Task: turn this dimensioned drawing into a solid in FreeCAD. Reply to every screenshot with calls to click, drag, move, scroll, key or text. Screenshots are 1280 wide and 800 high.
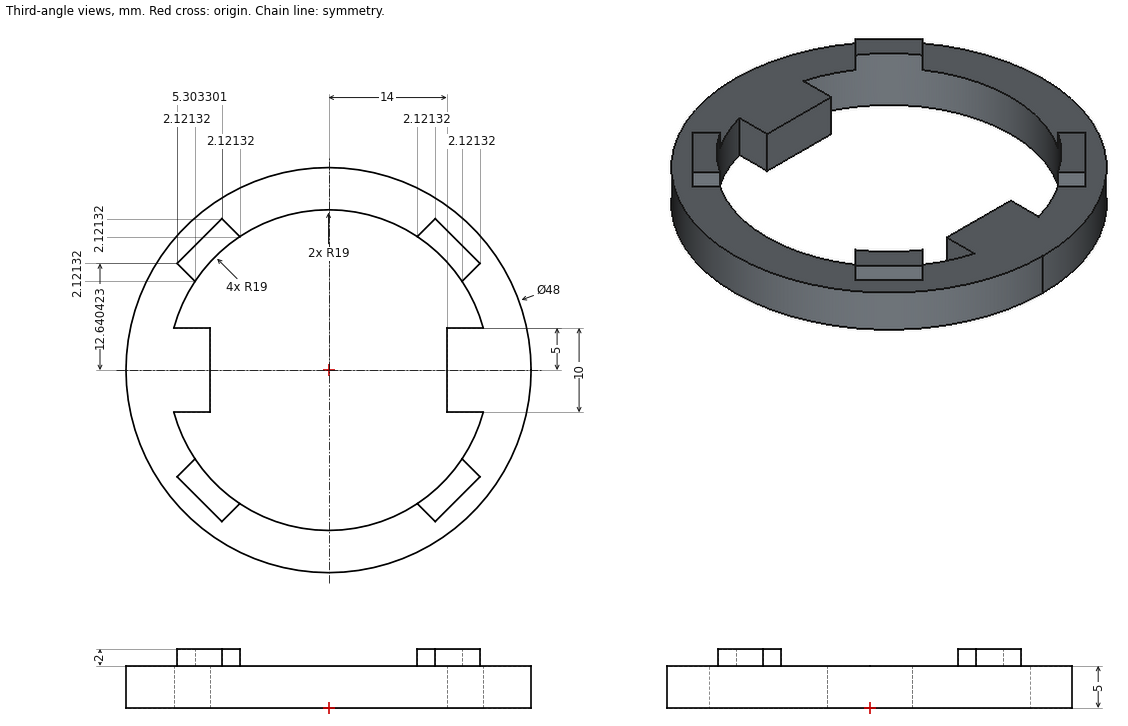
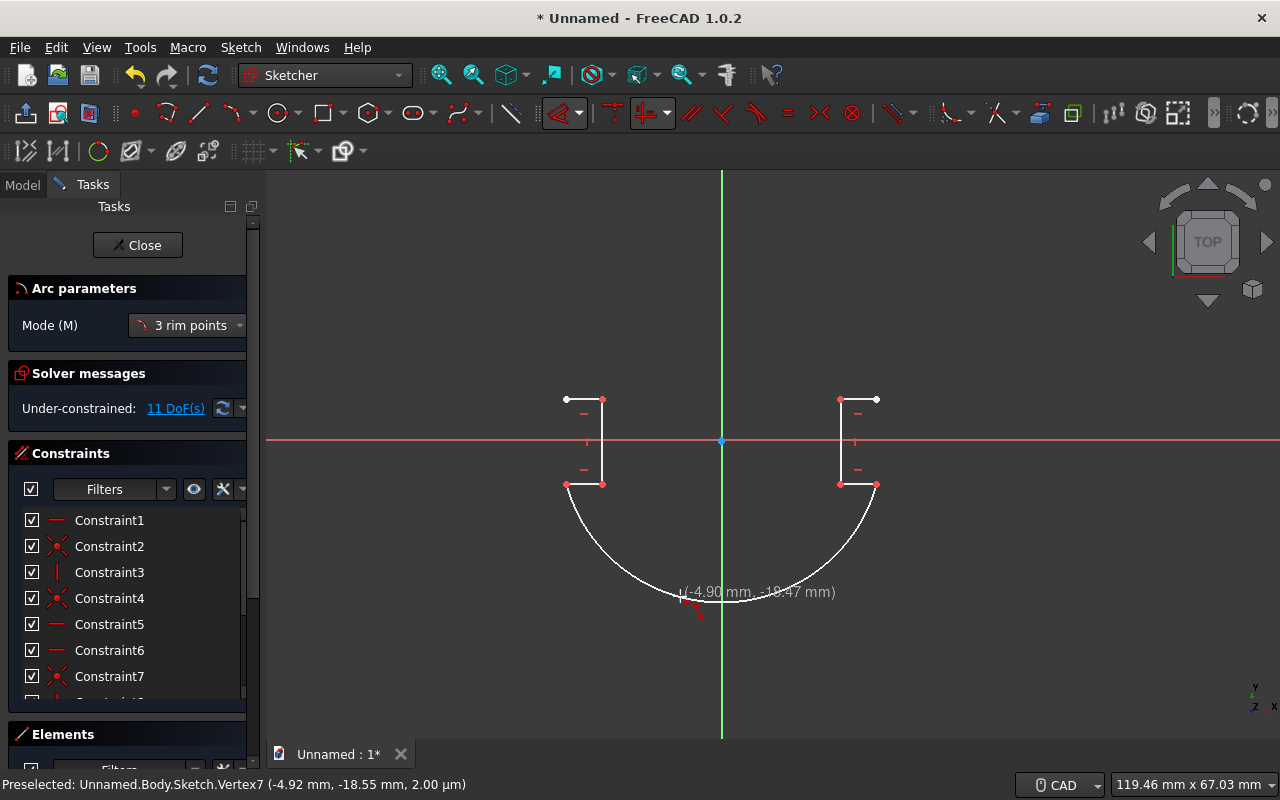
click(566, 399)
click(877, 399)
click(763, 284)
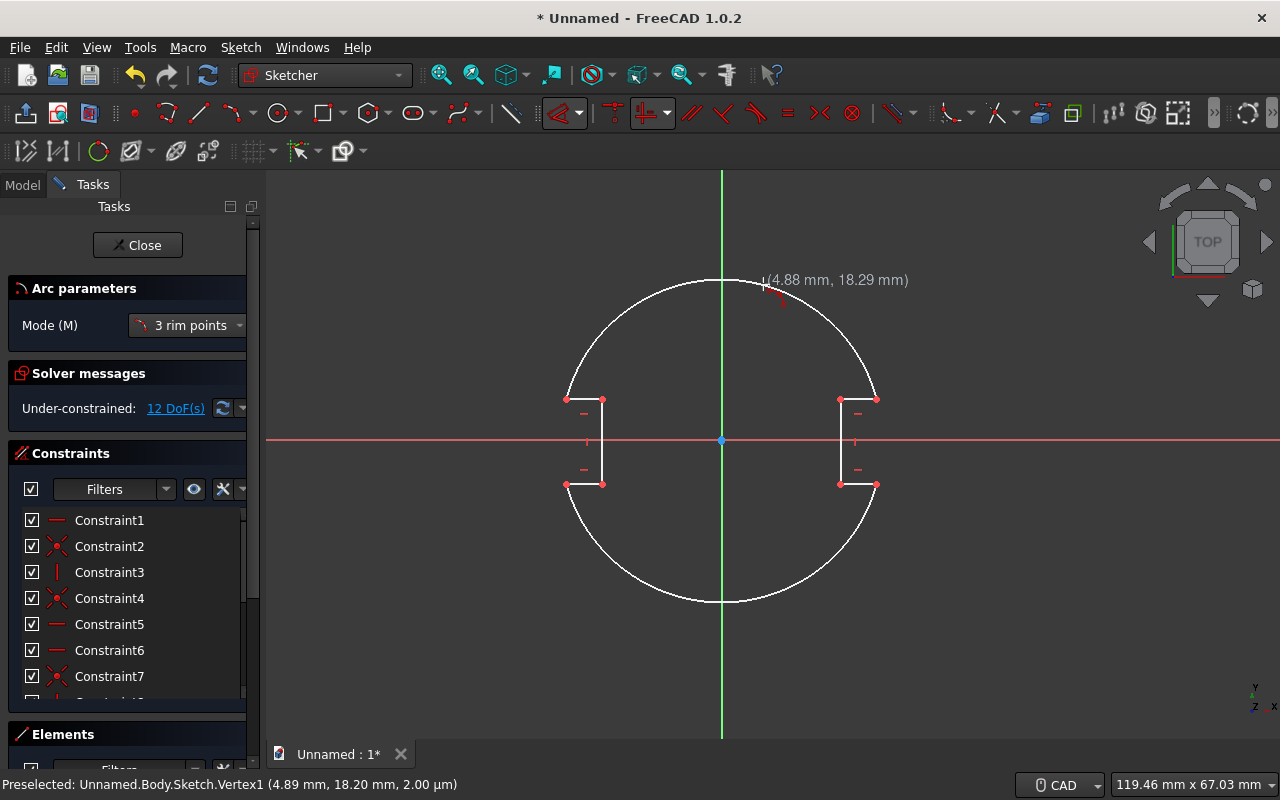
key(g)
key(c)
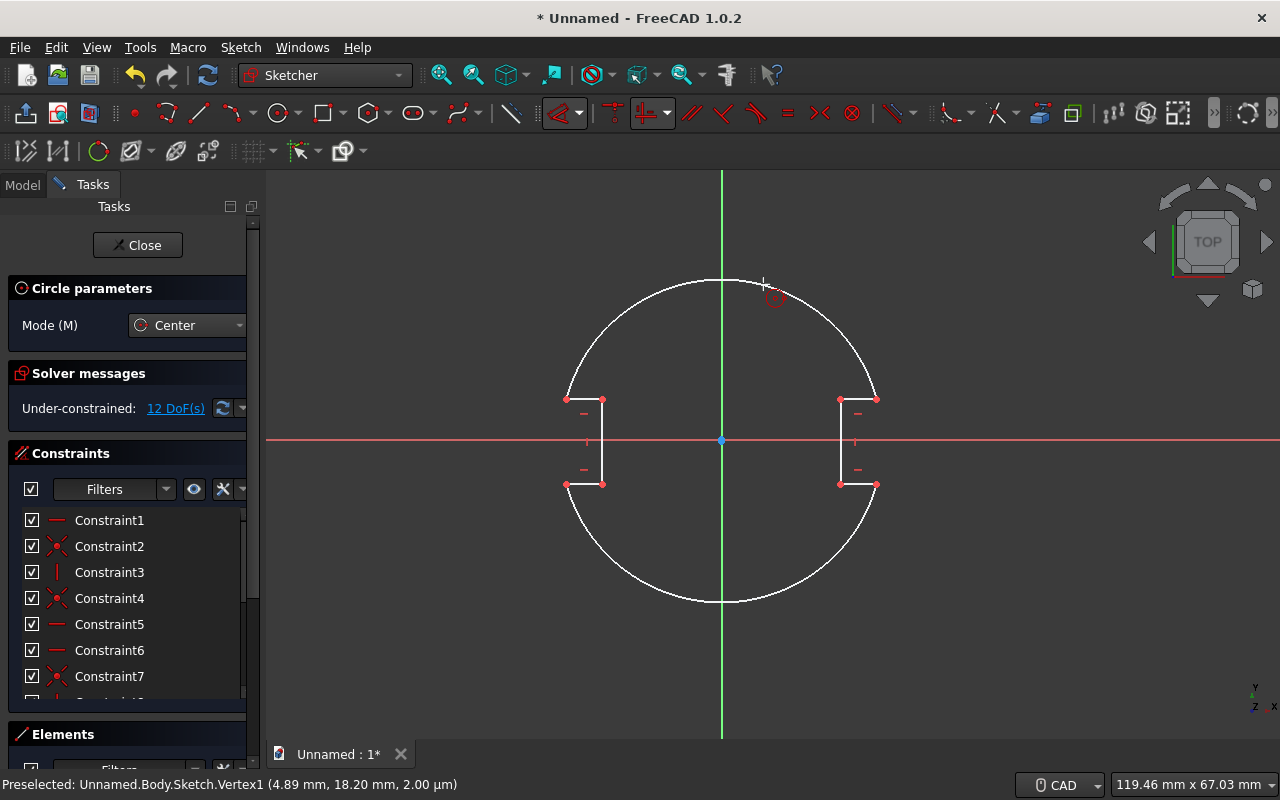
click(722, 440)
click(866, 296)
key(Escape)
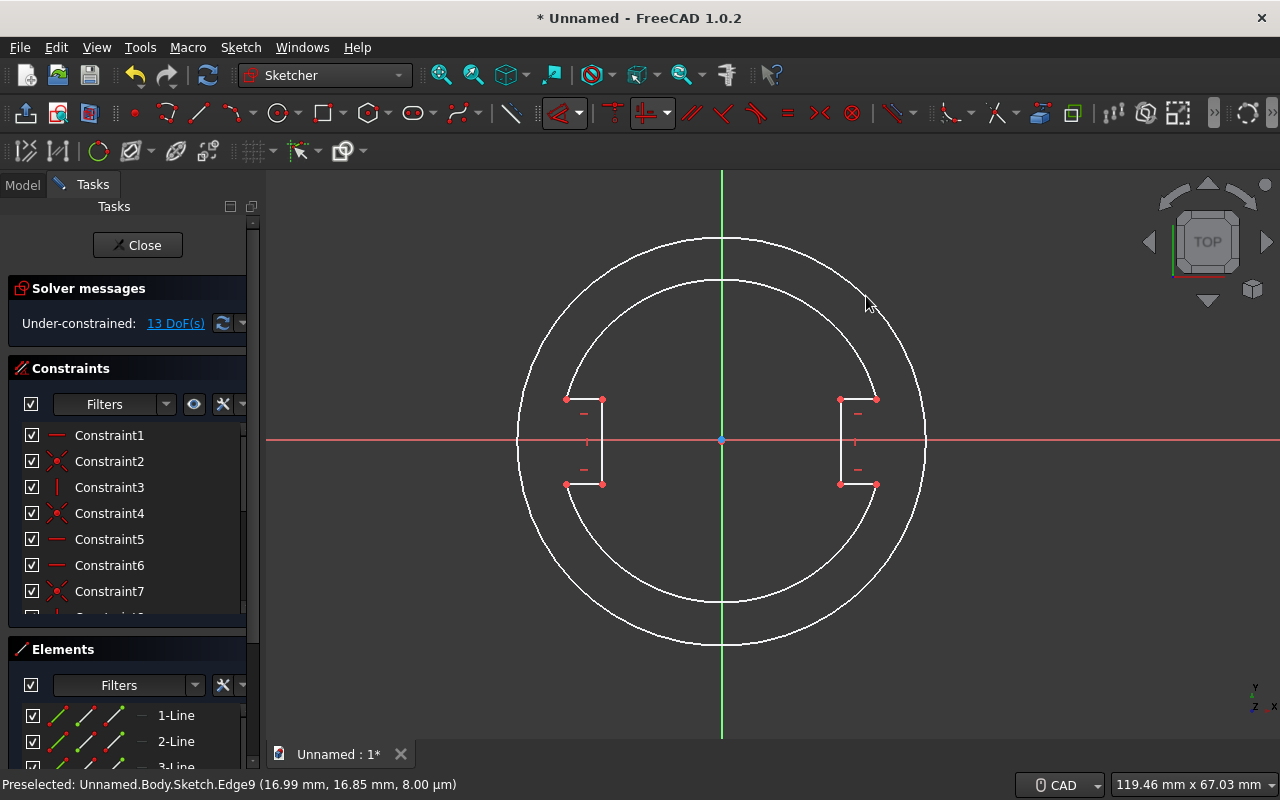
click(866, 297)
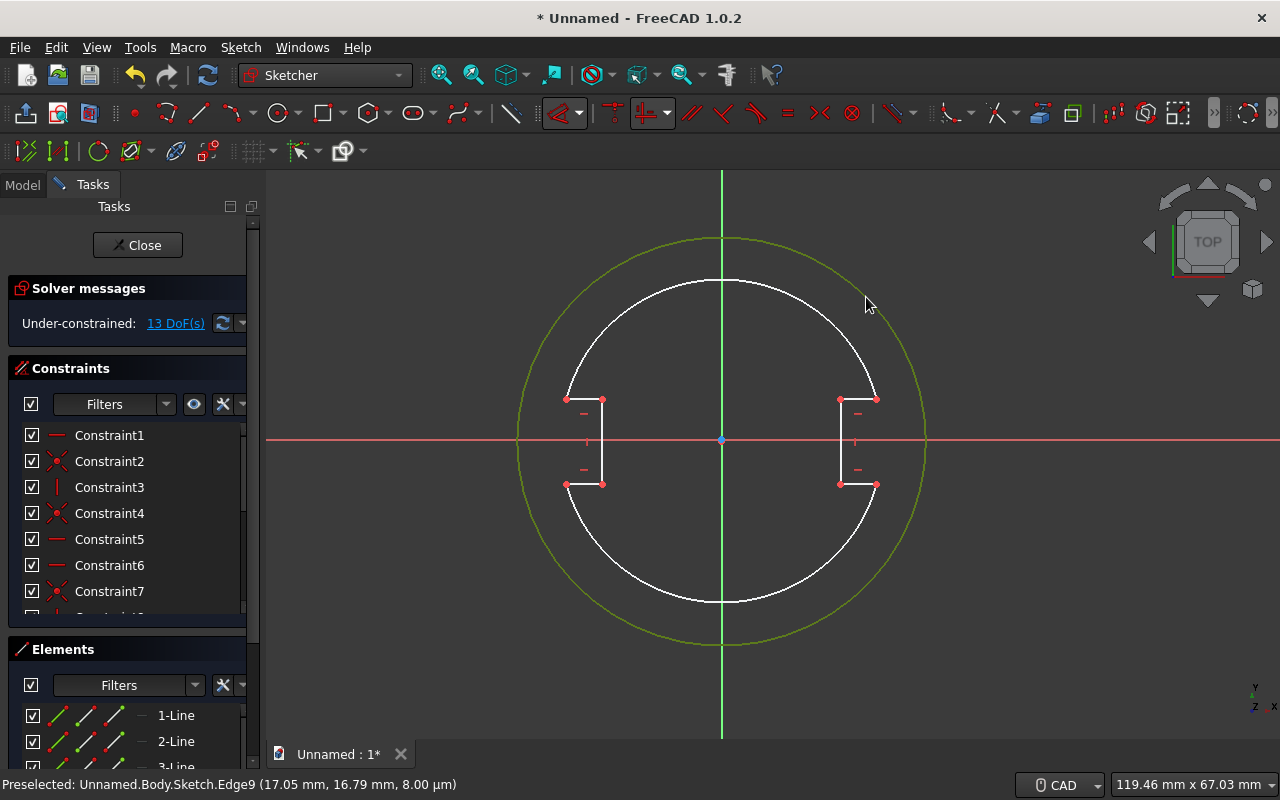
click(802, 301)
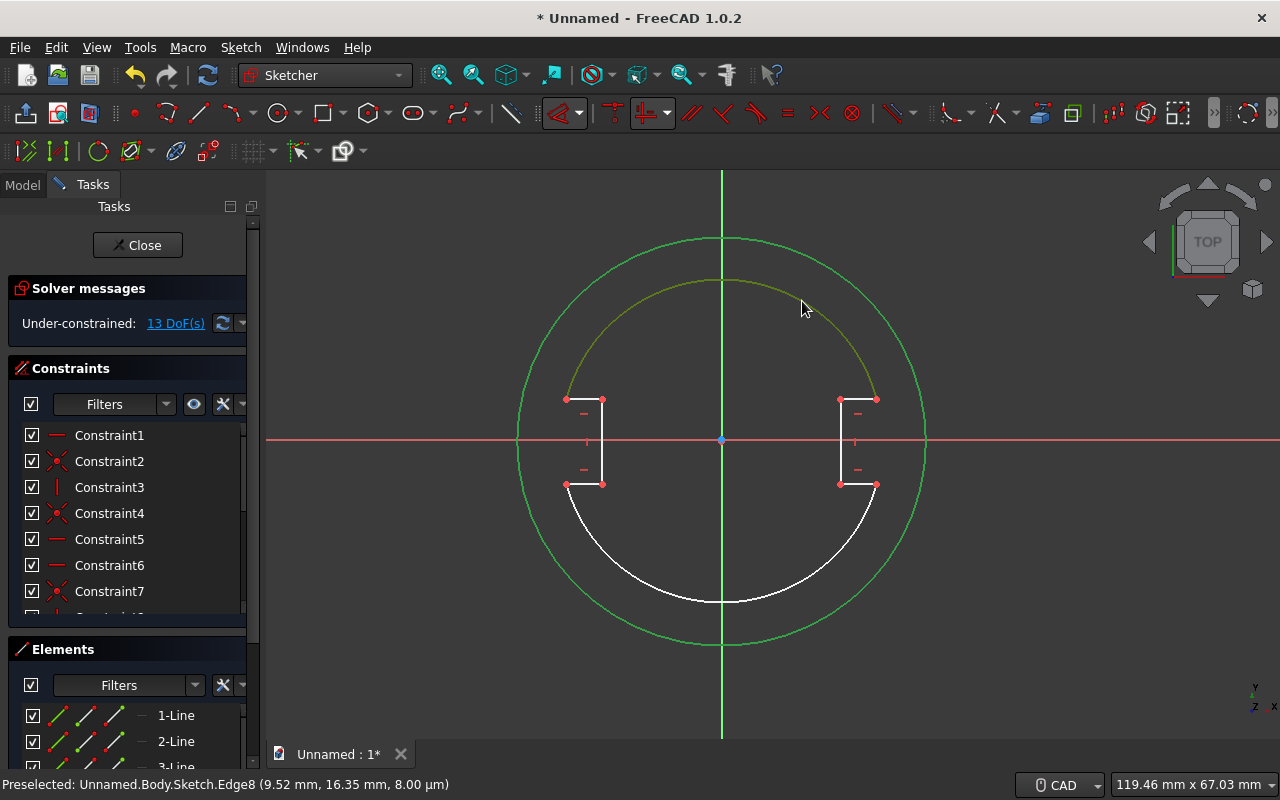
key(c)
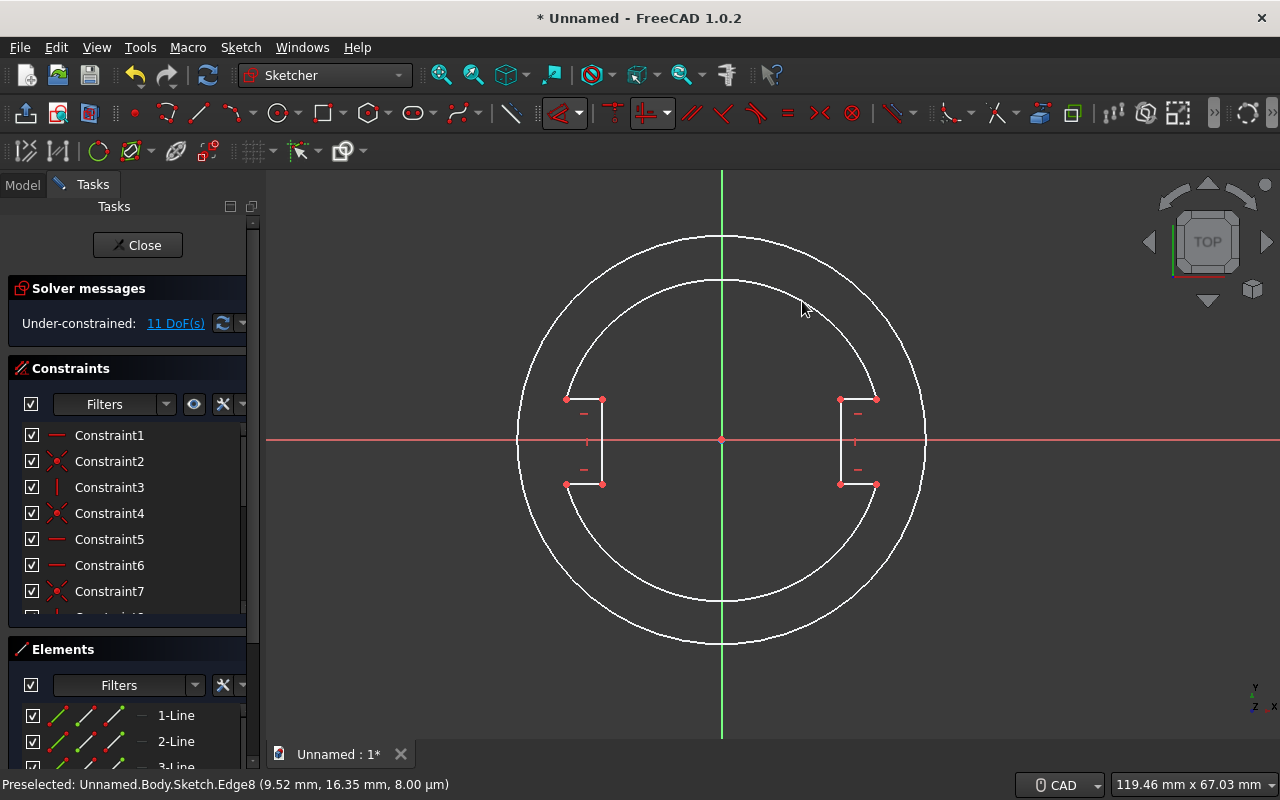
drag(712, 430, 732, 450)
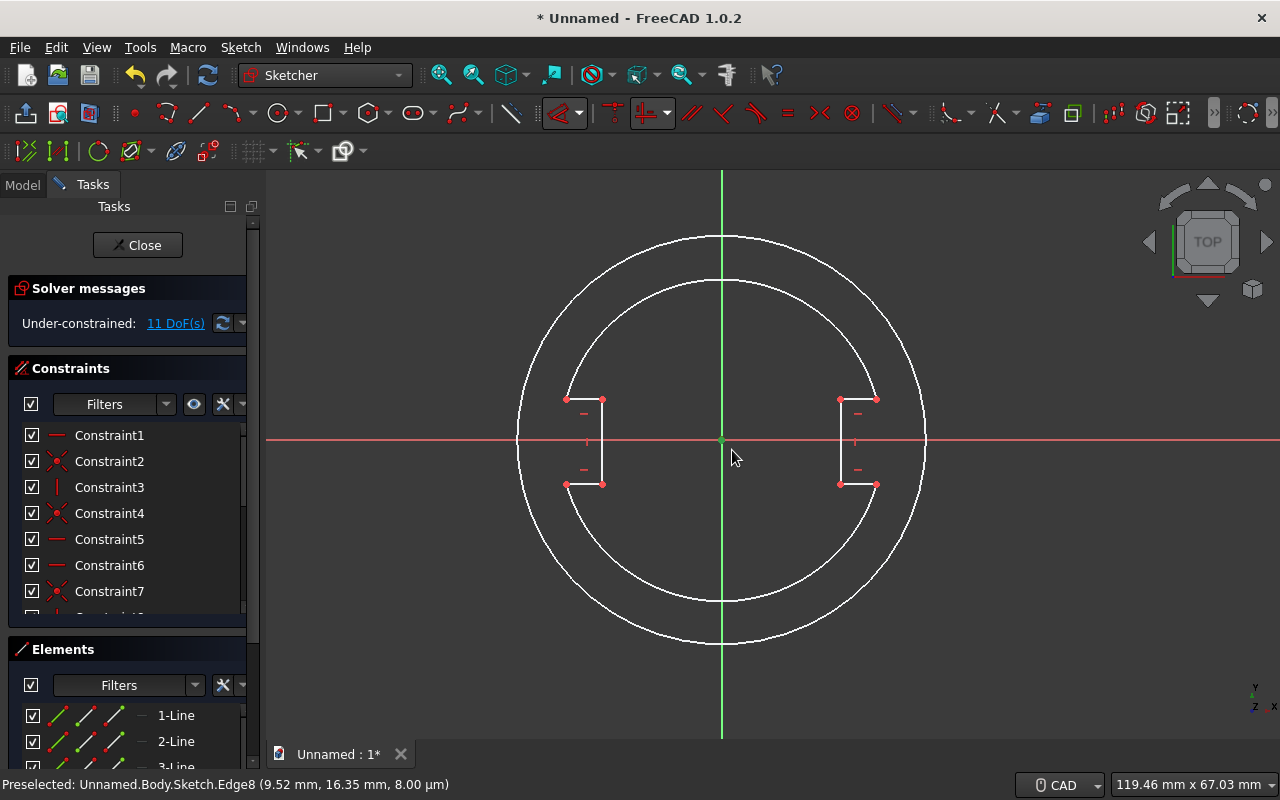
key(c)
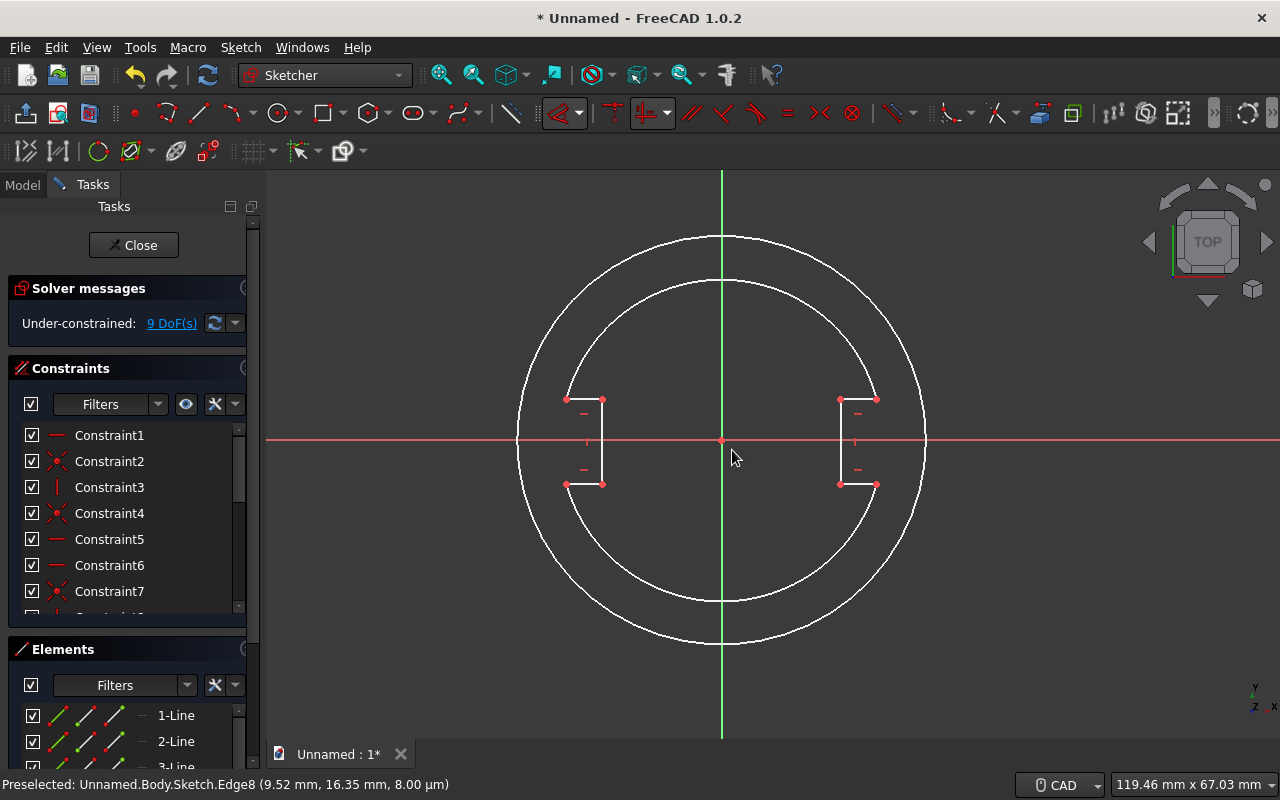
click(642, 580)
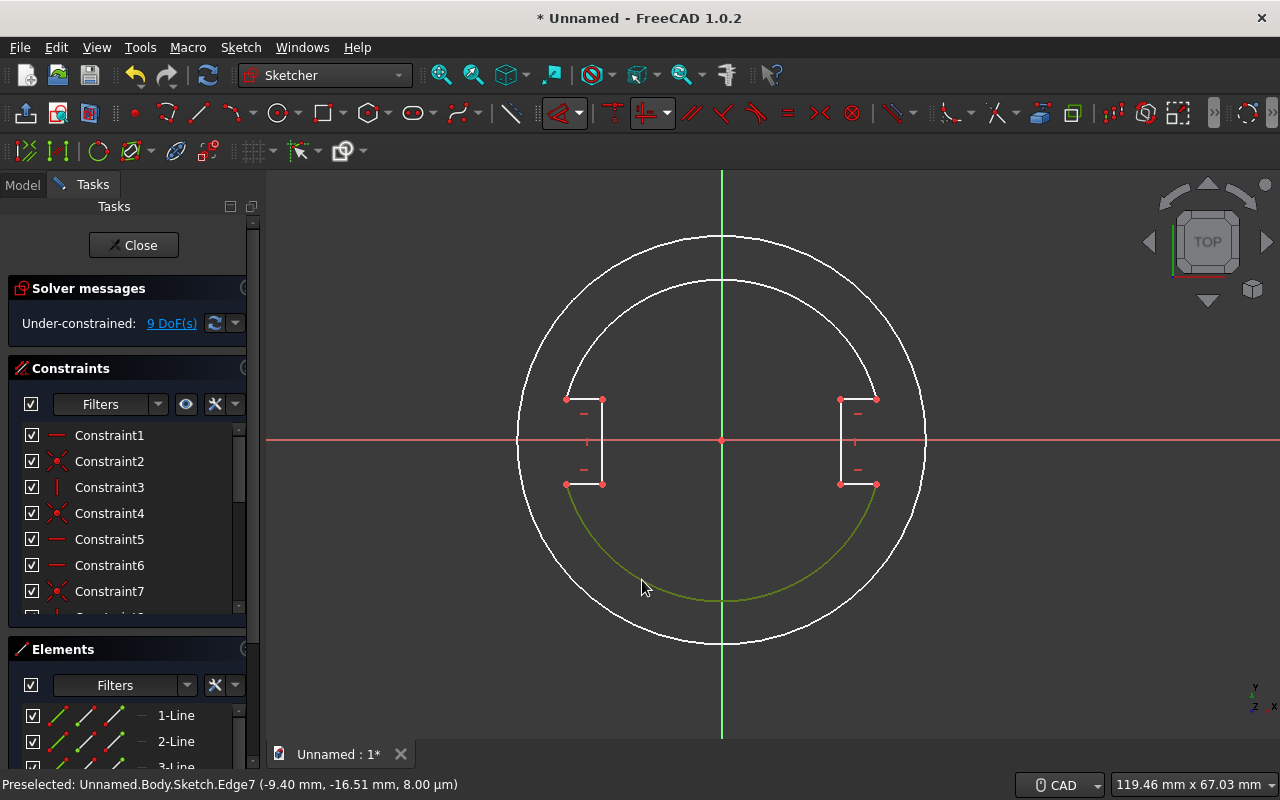
click(802, 301)